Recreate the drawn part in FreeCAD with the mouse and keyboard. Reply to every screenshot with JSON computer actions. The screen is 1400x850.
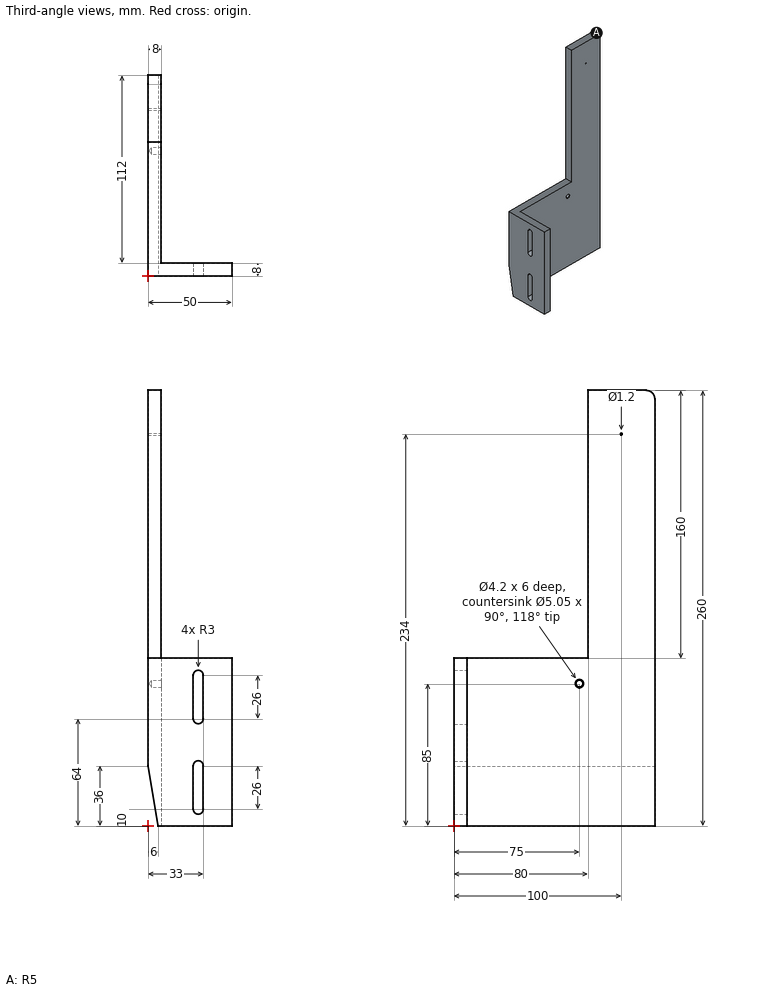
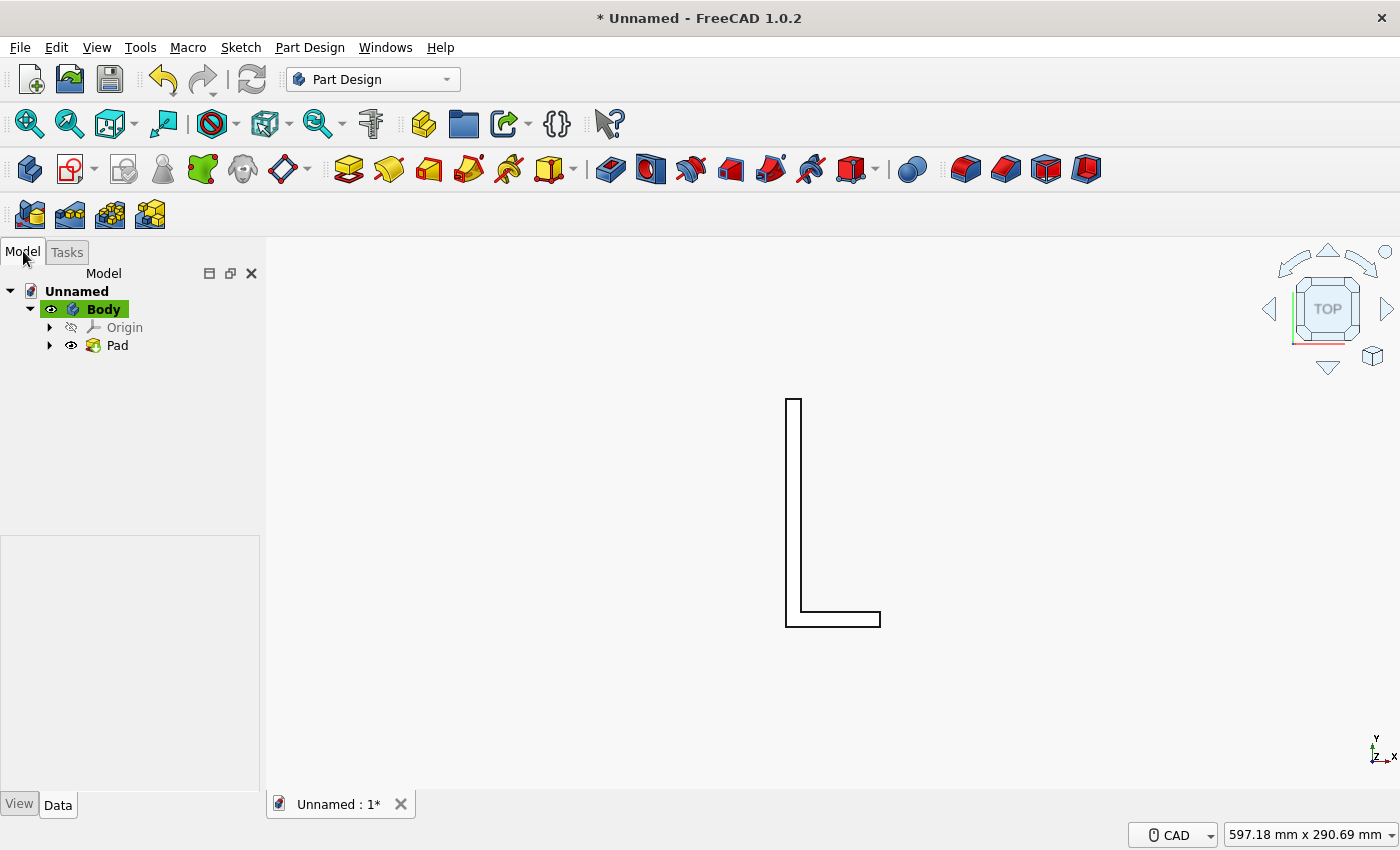
{"action": "left_click", "coordinate": [50, 327]}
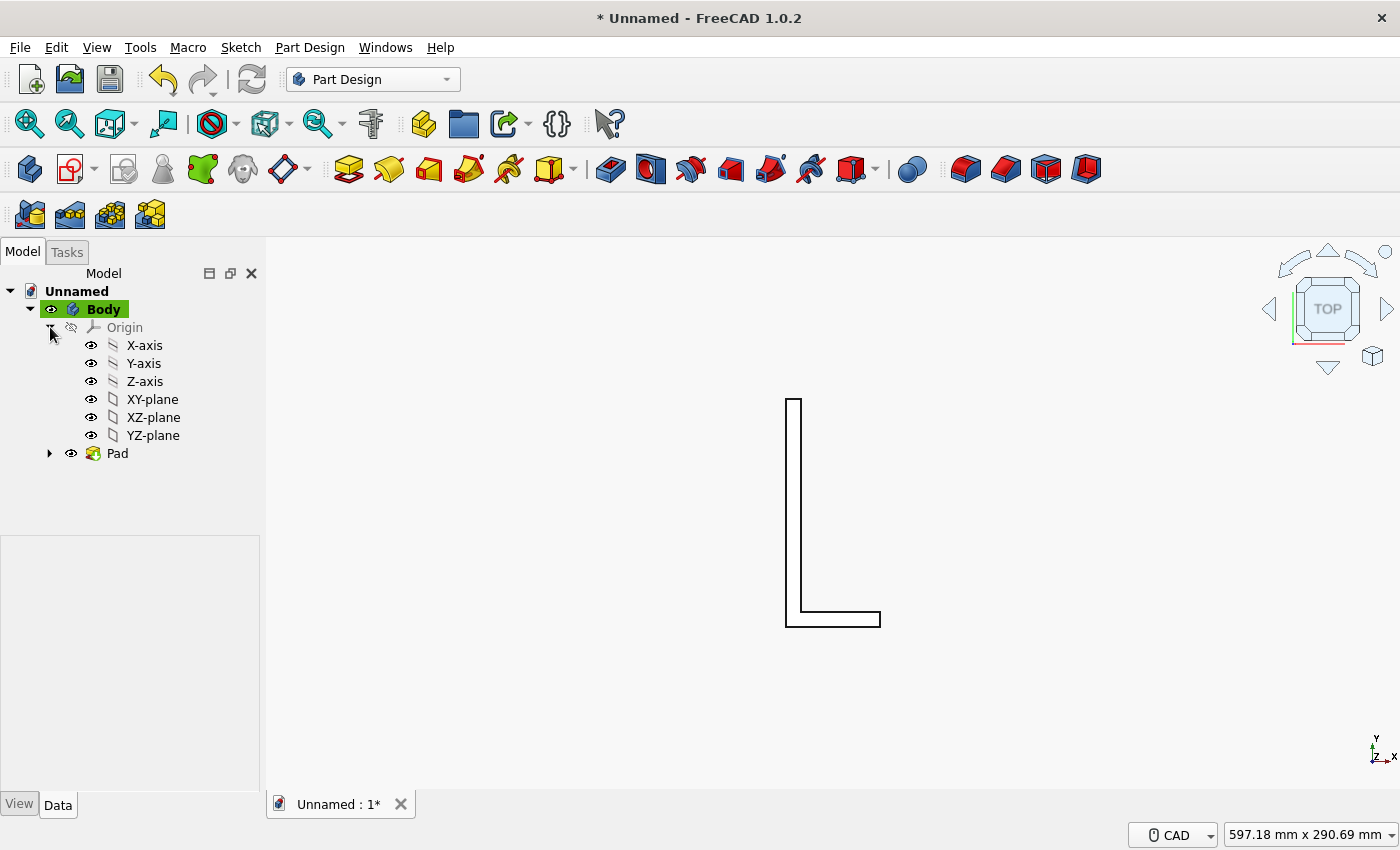
{"action": "left_click", "coordinate": [136, 435]}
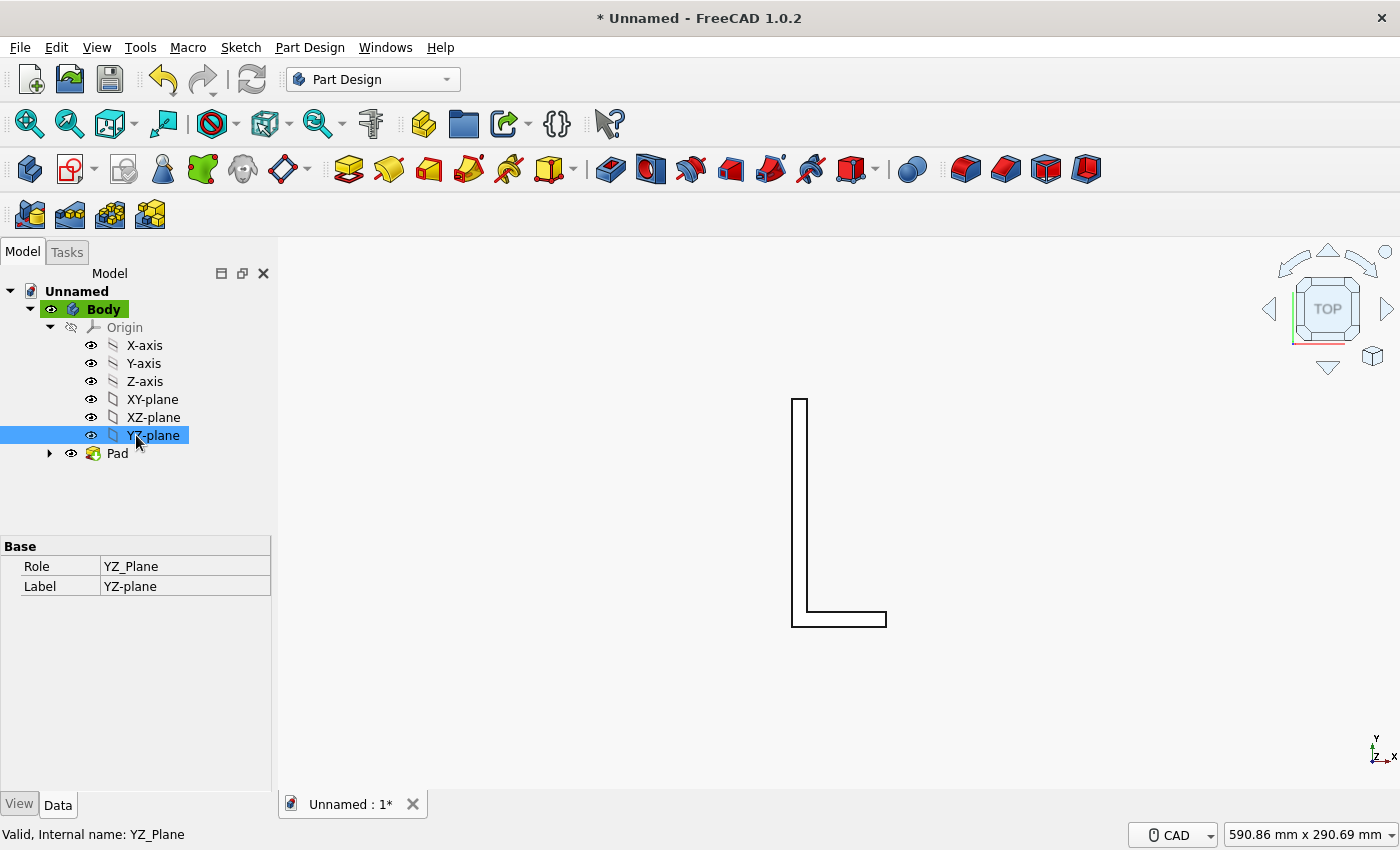
{"action": "left_click", "coordinate": [284, 170]}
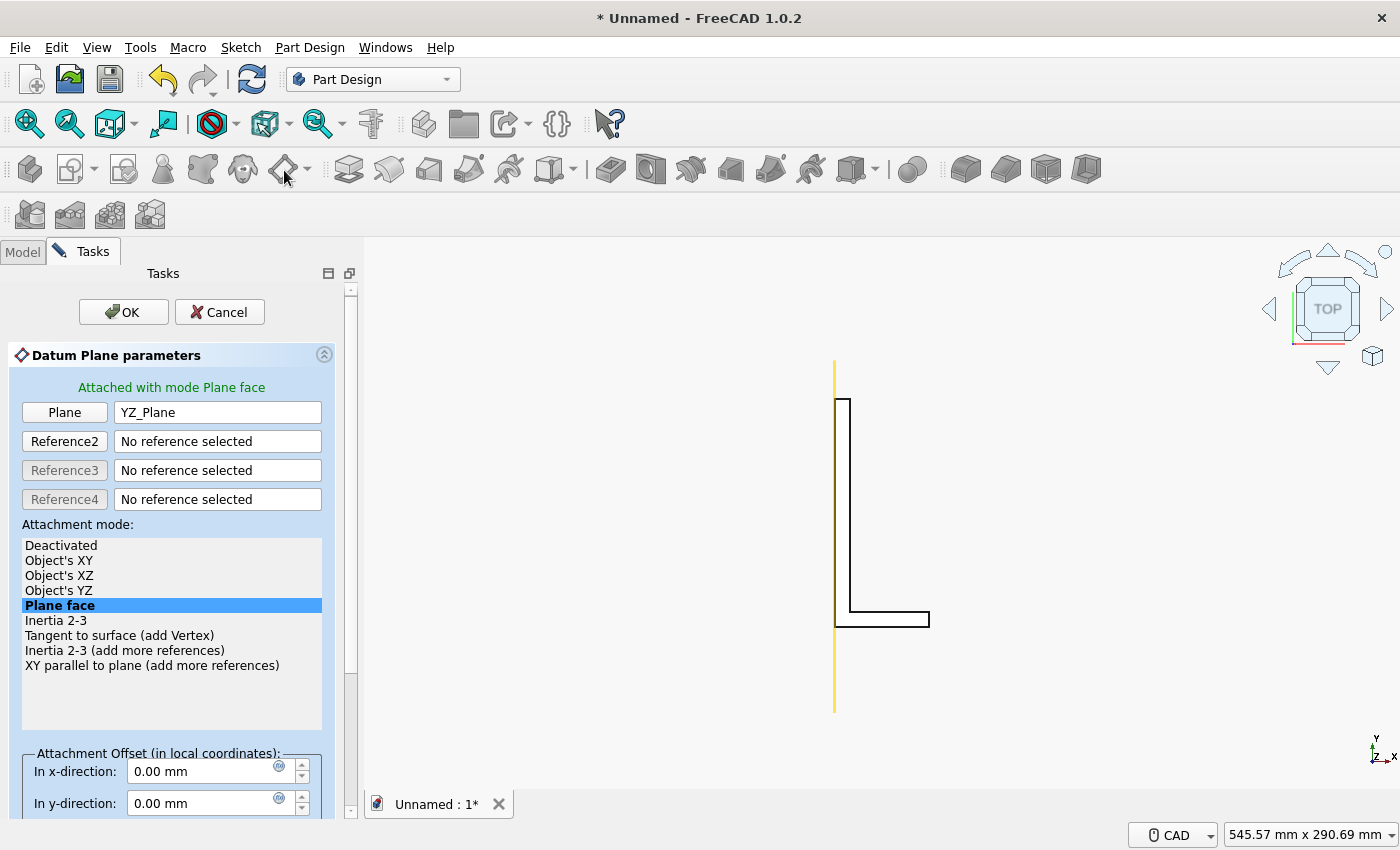
{"action": "scroll", "coordinate": [351, 550], "scroll_direction": "down", "scroll_amount": 2}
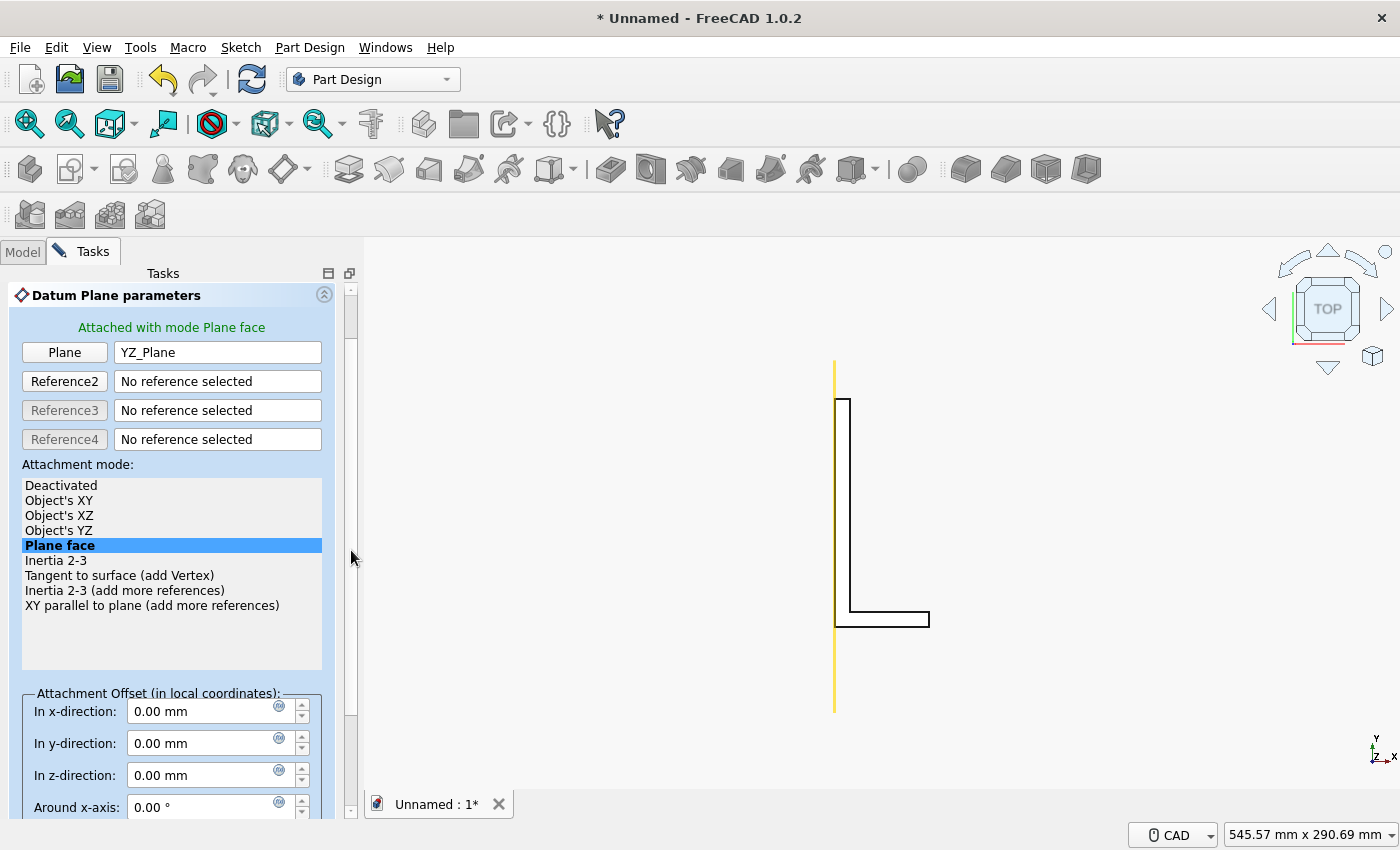
{"action": "triple_click", "coordinate": [210, 715]}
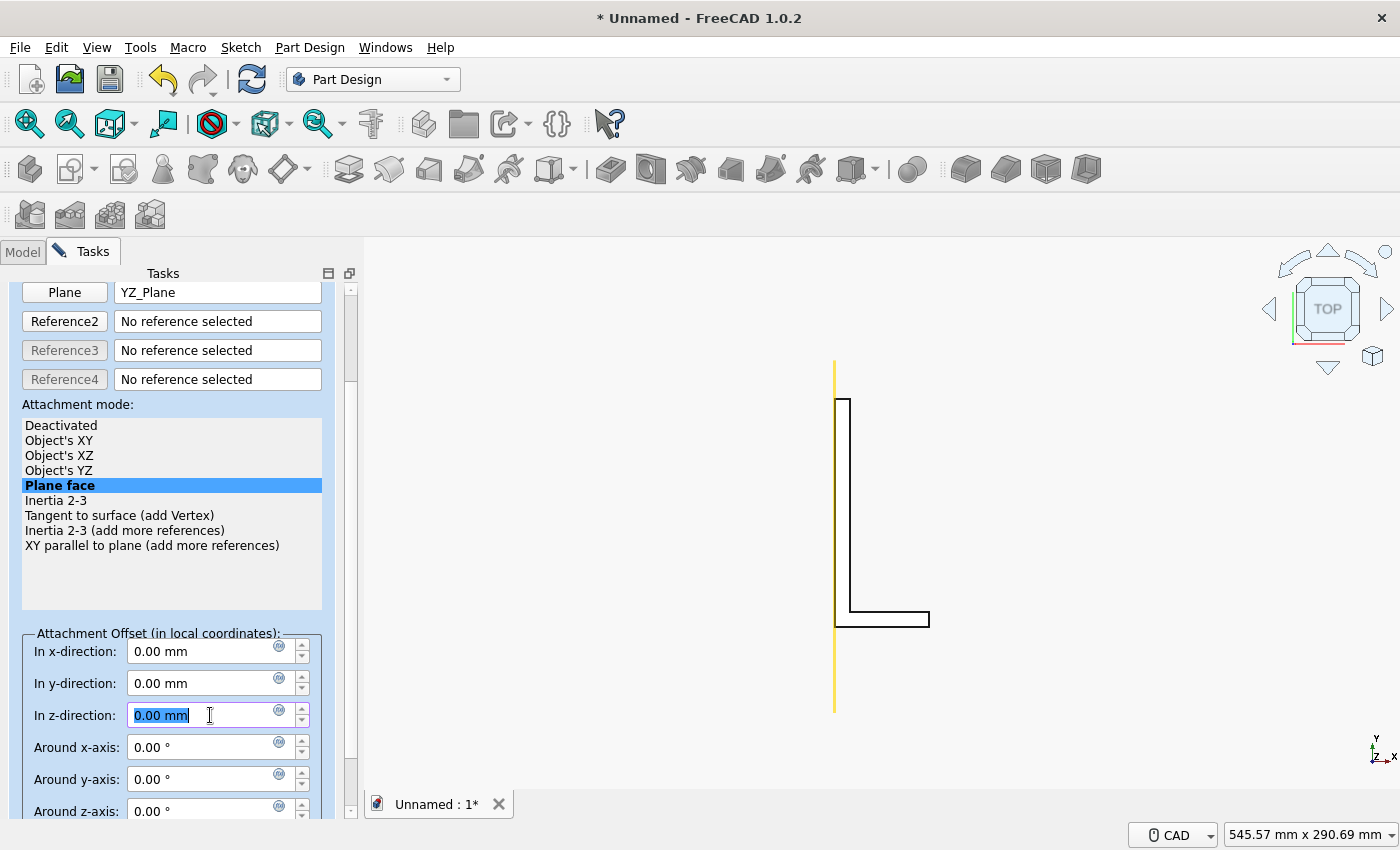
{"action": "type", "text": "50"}
{"action": "key", "text": "Tab"}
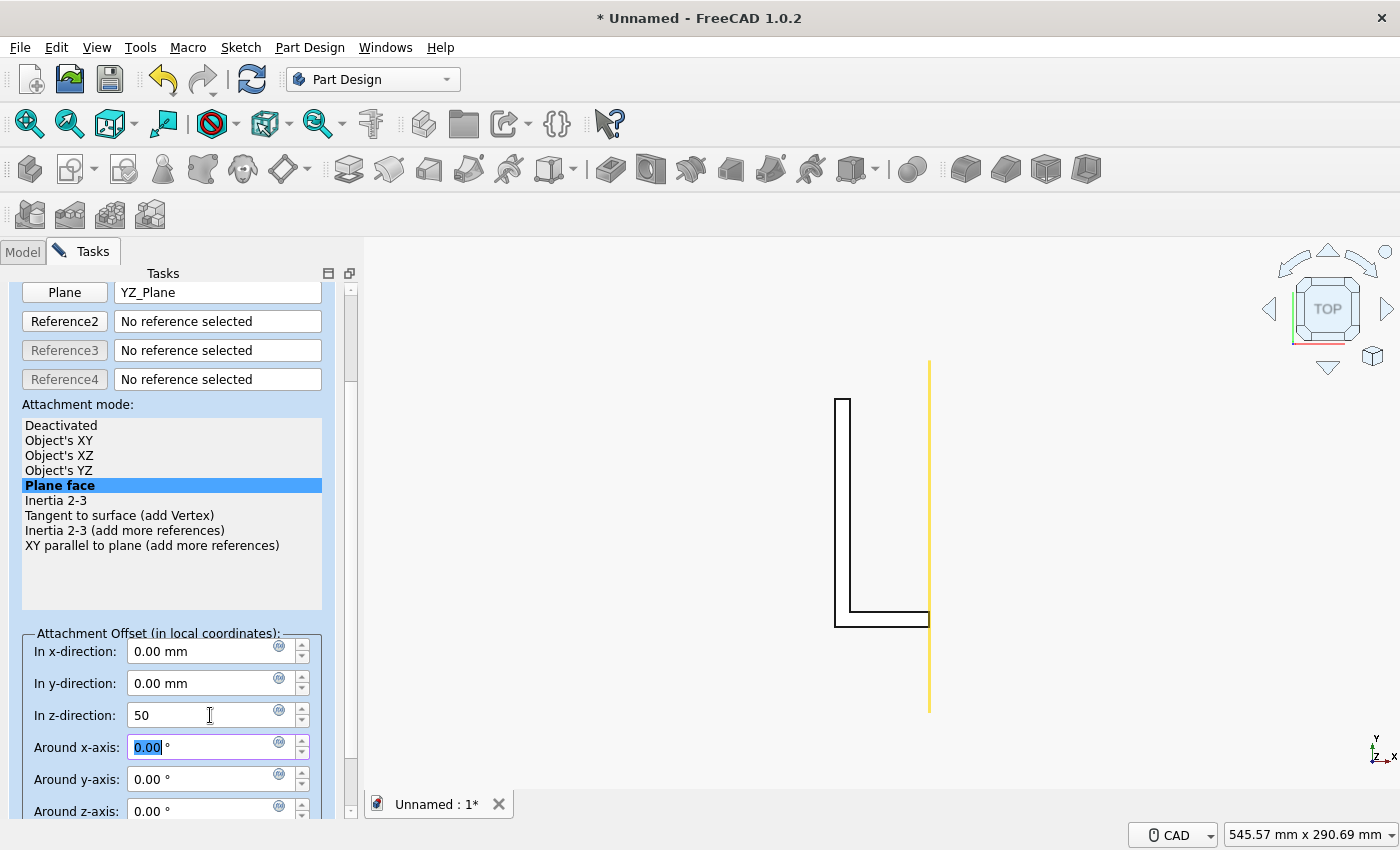
{"action": "scroll", "coordinate": [351, 550], "scroll_direction": "up", "scroll_amount": 3}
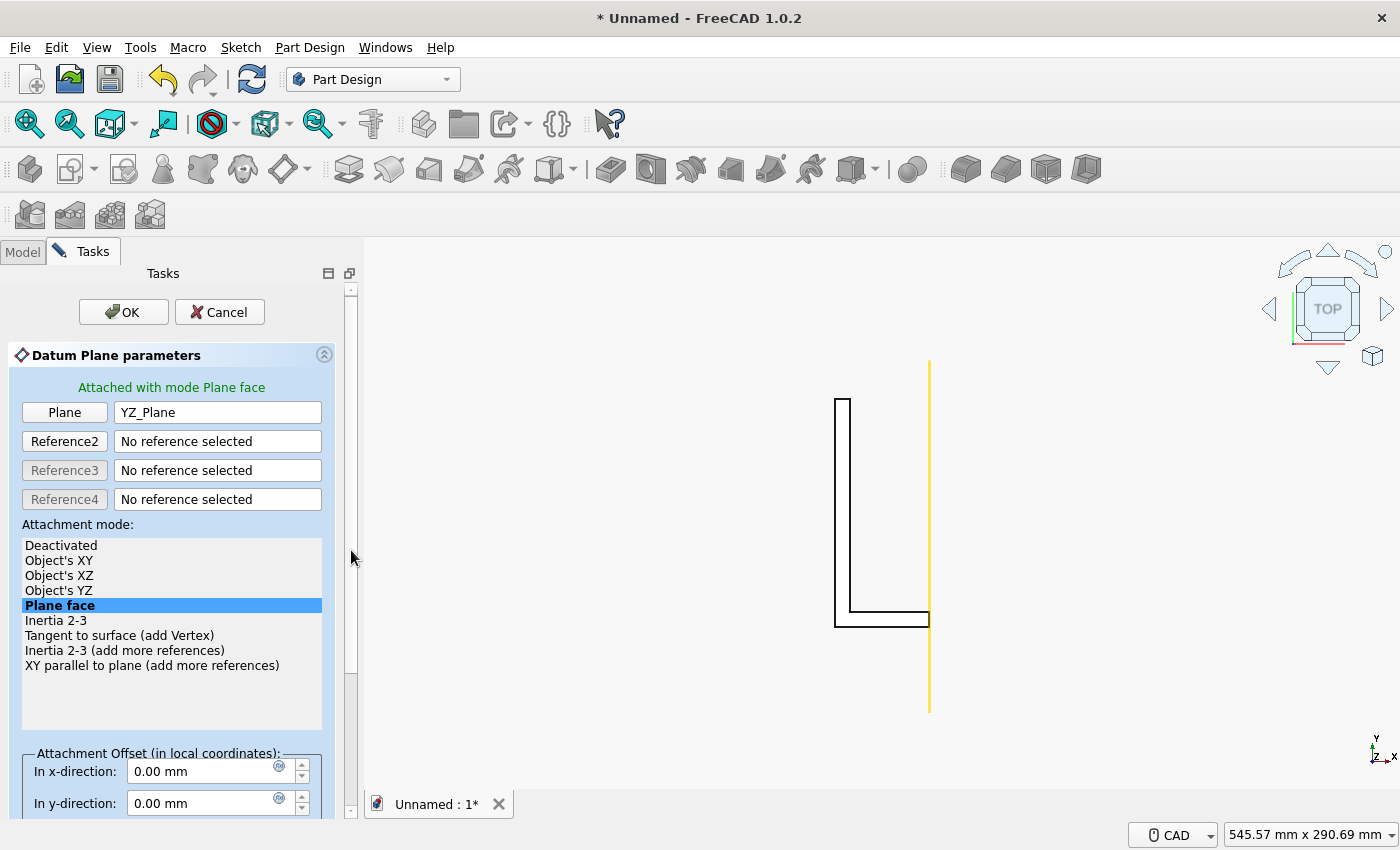
{"action": "left_click", "coordinate": [124, 312]}